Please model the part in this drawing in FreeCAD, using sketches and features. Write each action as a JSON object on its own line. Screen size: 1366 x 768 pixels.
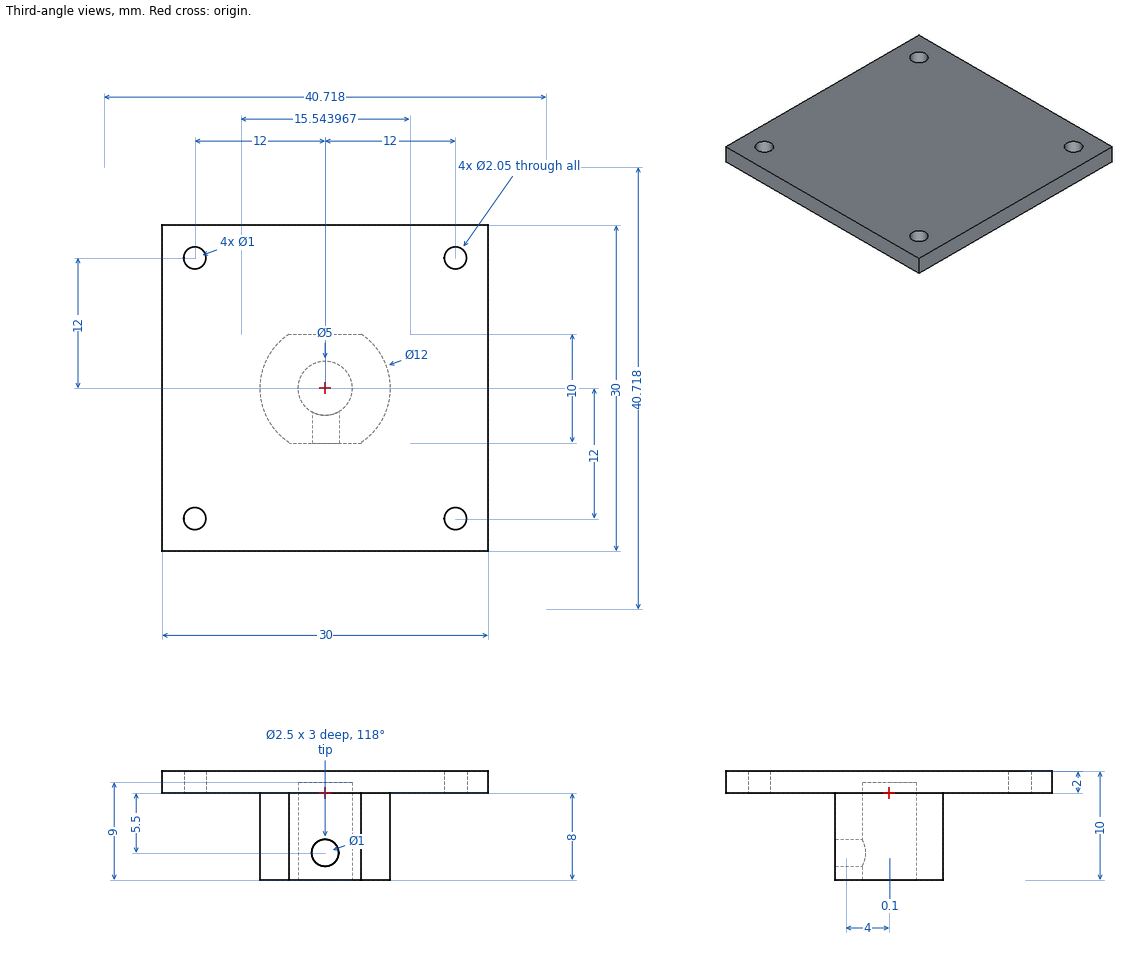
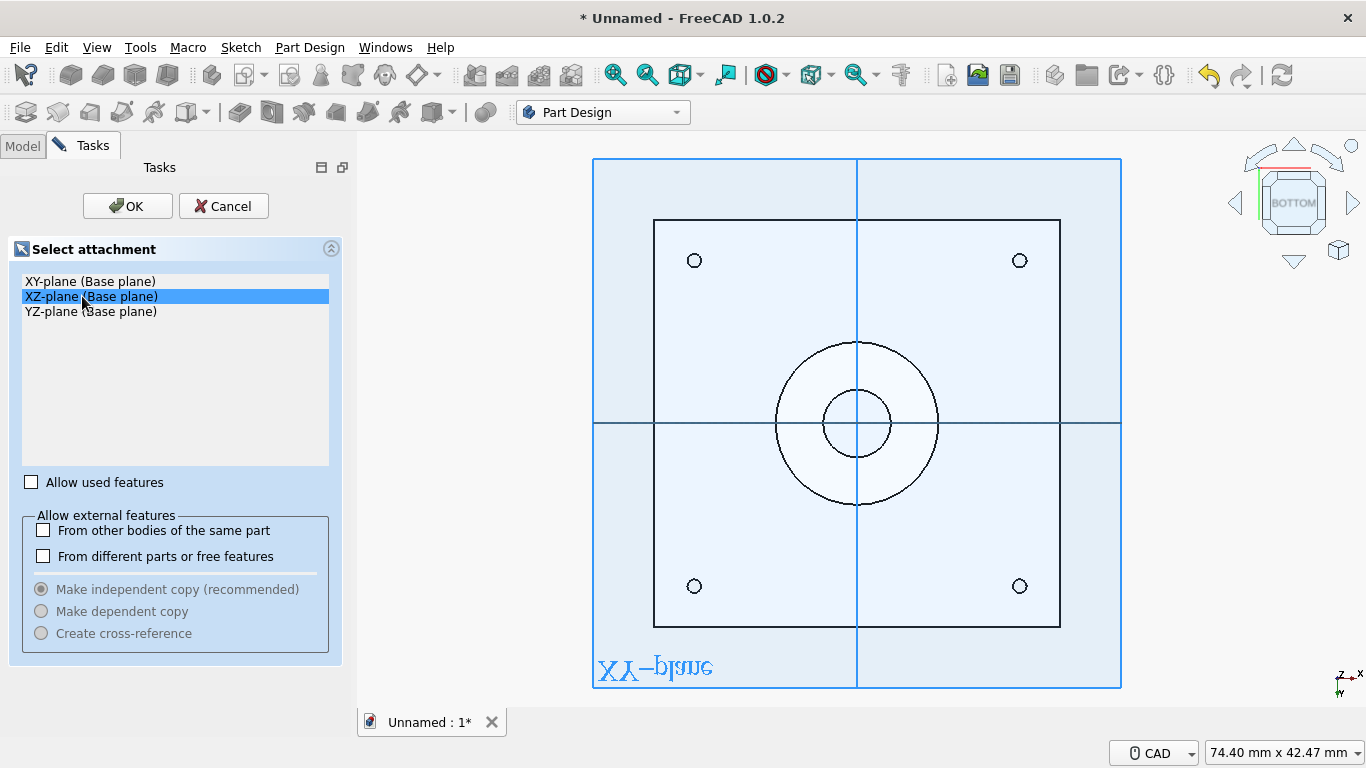
{"action": "left_click", "coordinate": [128, 206]}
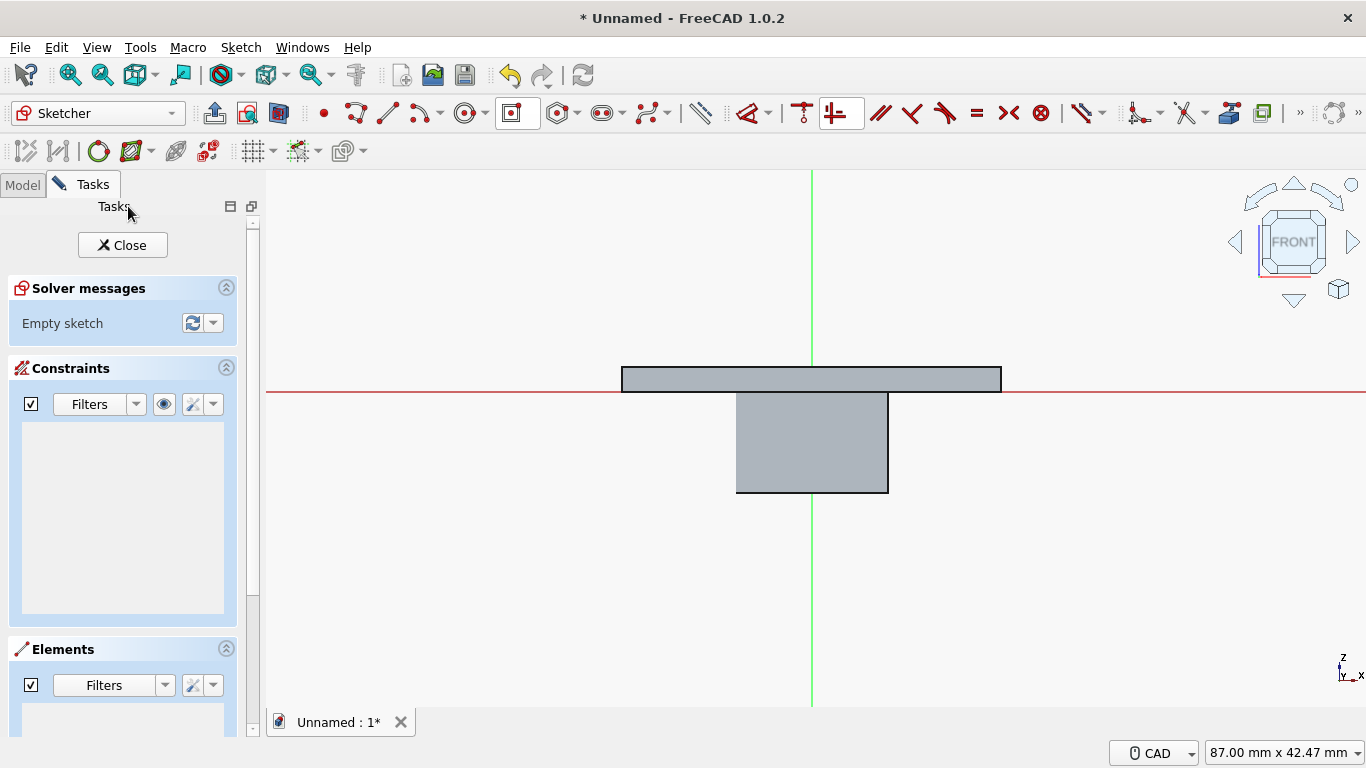
{"action": "key", "text": "q s"}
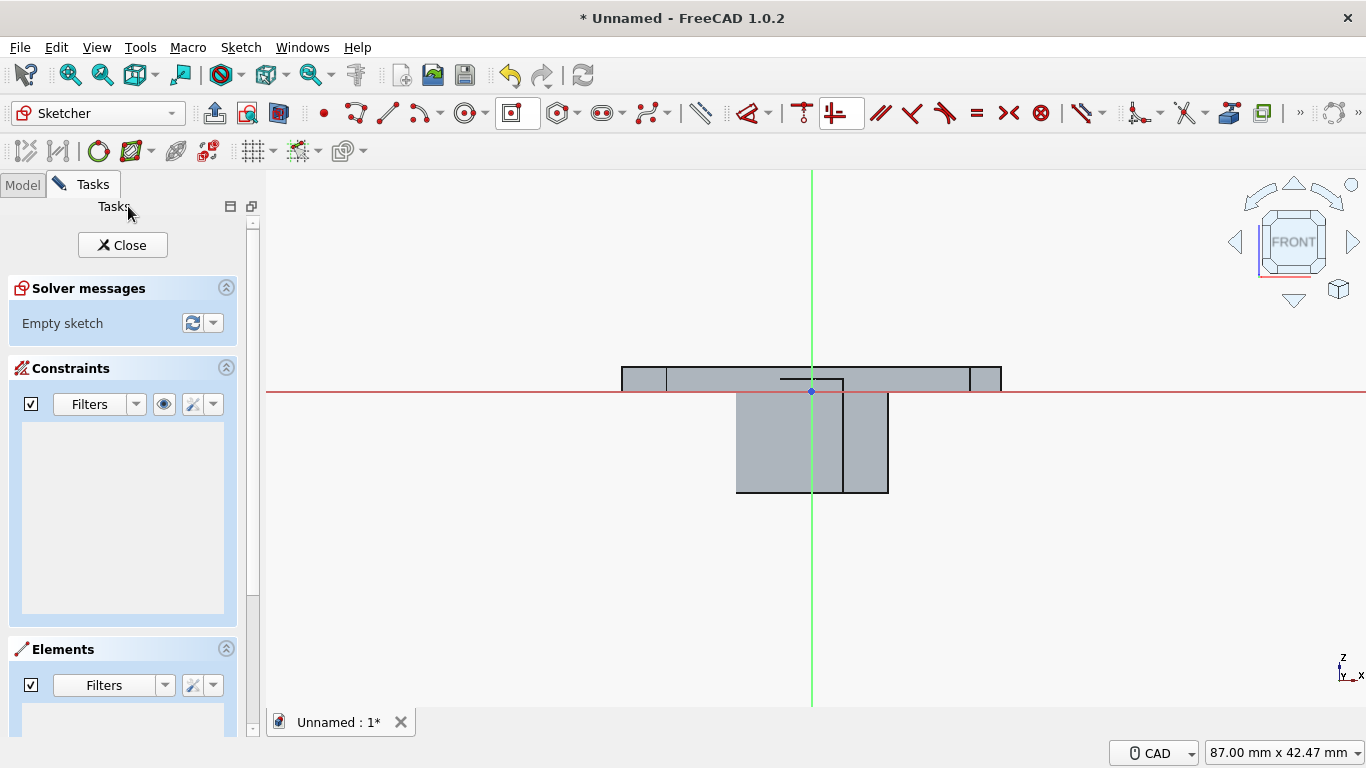
{"action": "scroll", "coordinate": [815, 463], "scroll_direction": "up", "scroll_amount": 15}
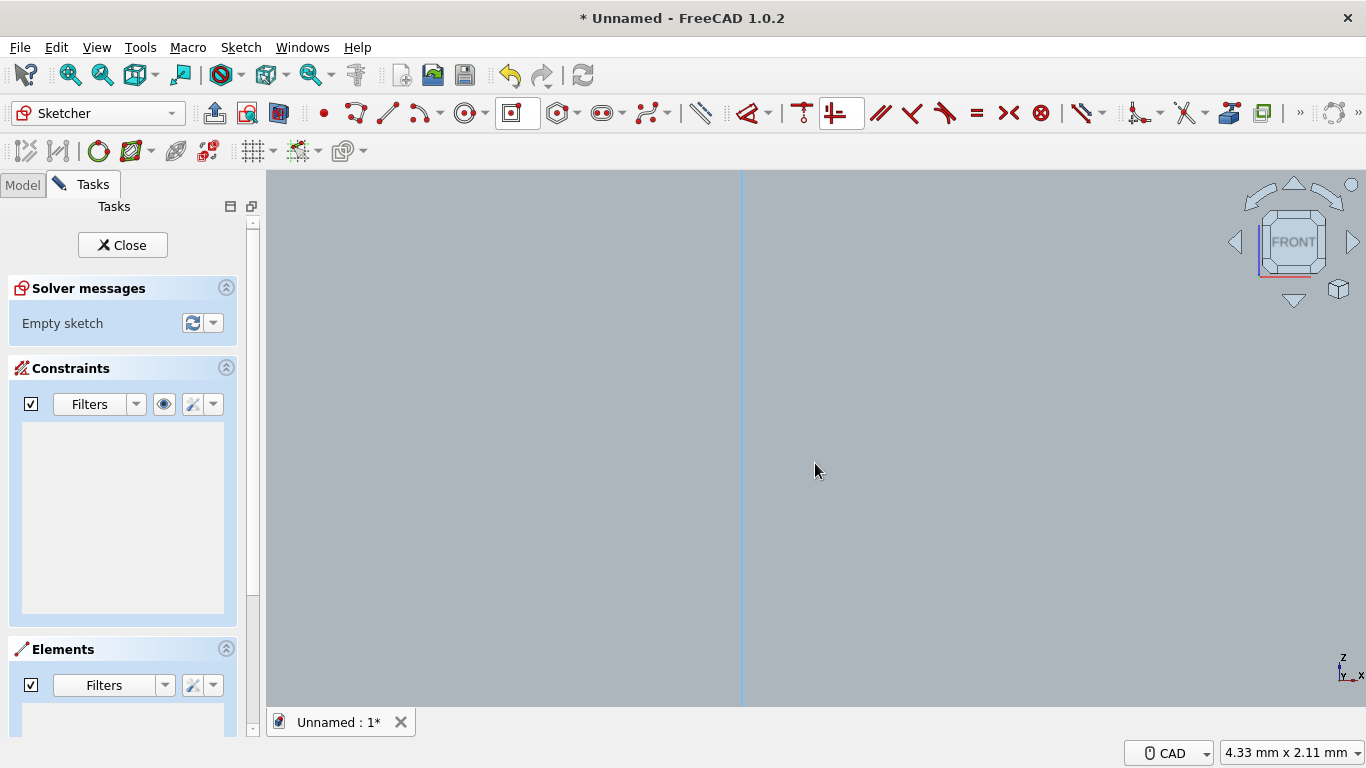
{"action": "key", "text": "g c"}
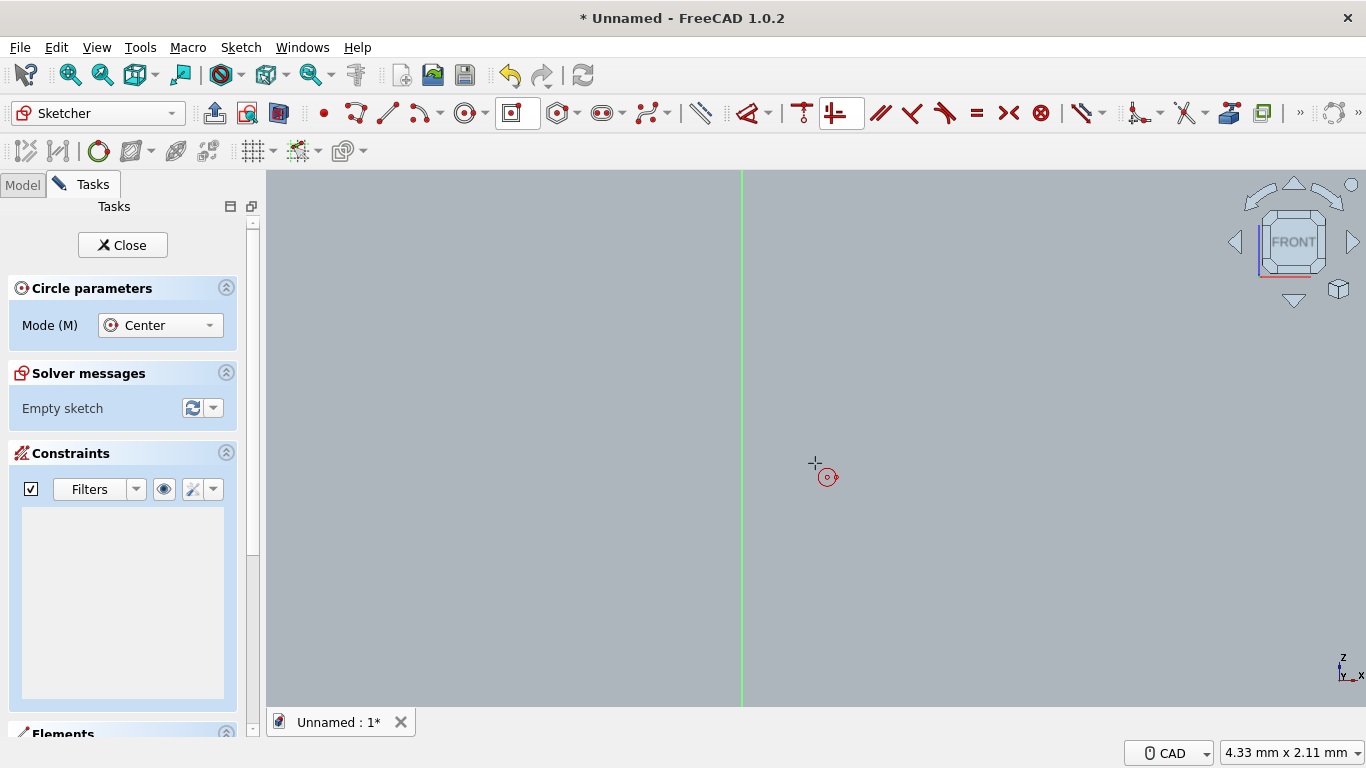
{"action": "left_click", "coordinate": [742, 421]}
{"action": "left_click", "coordinate": [832, 331]}
{"action": "key", "text": "Escape"}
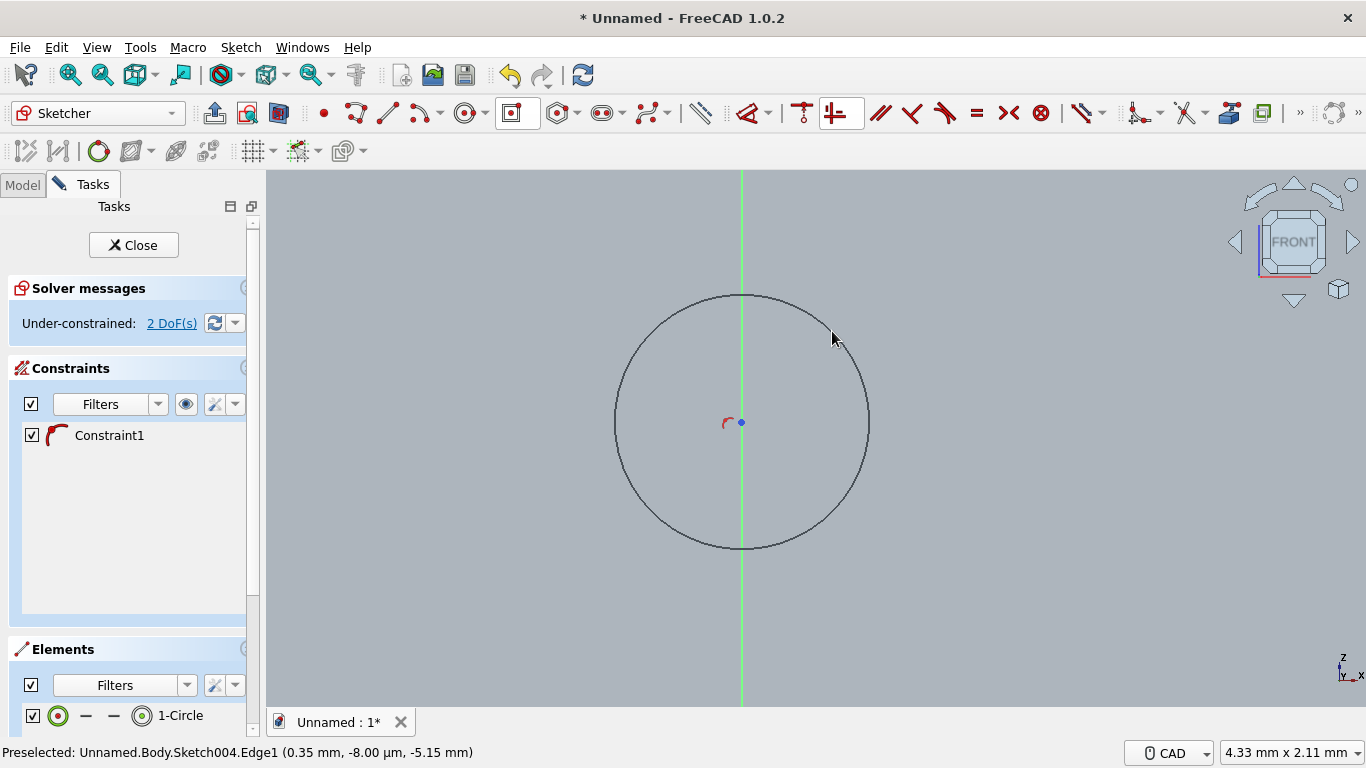
{"action": "left_click", "coordinate": [748, 114]}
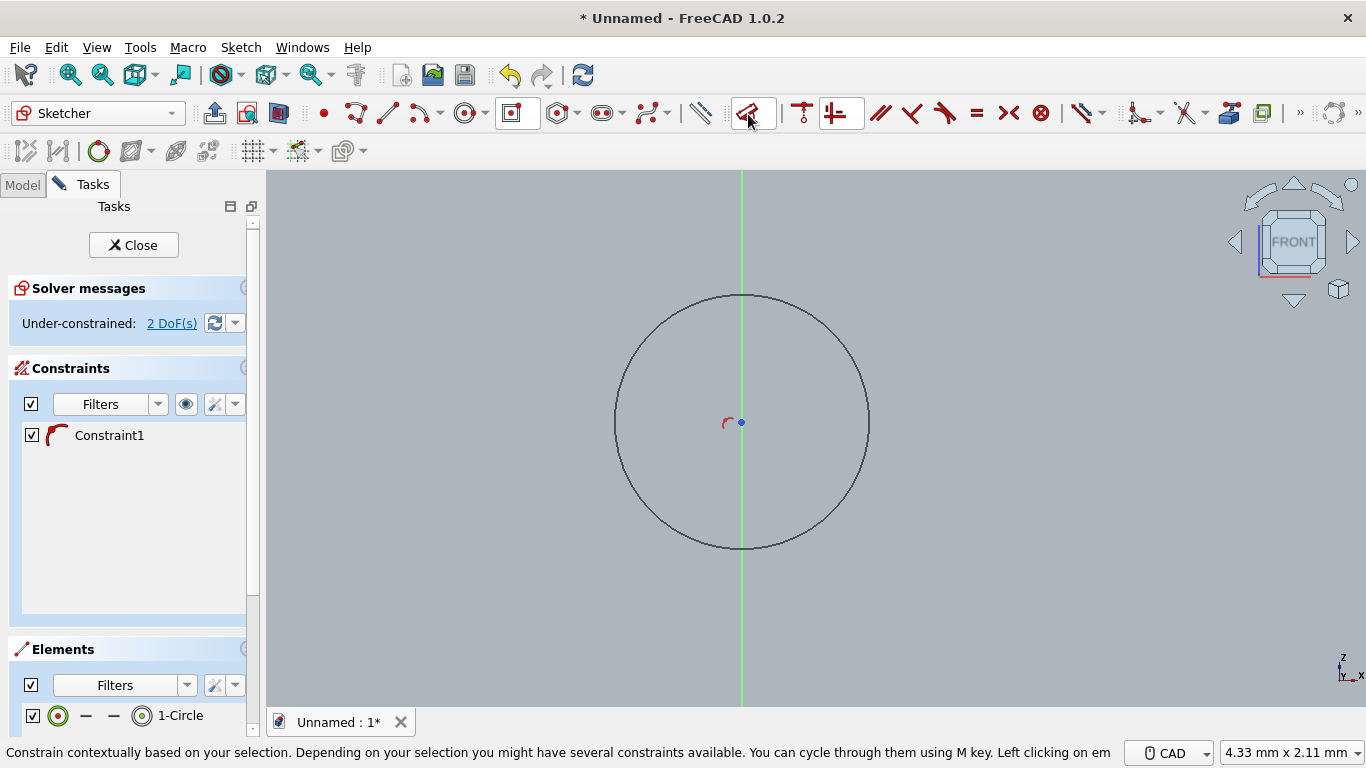
{"action": "left_click", "coordinate": [832, 332]}
{"action": "left_click", "coordinate": [855, 309]}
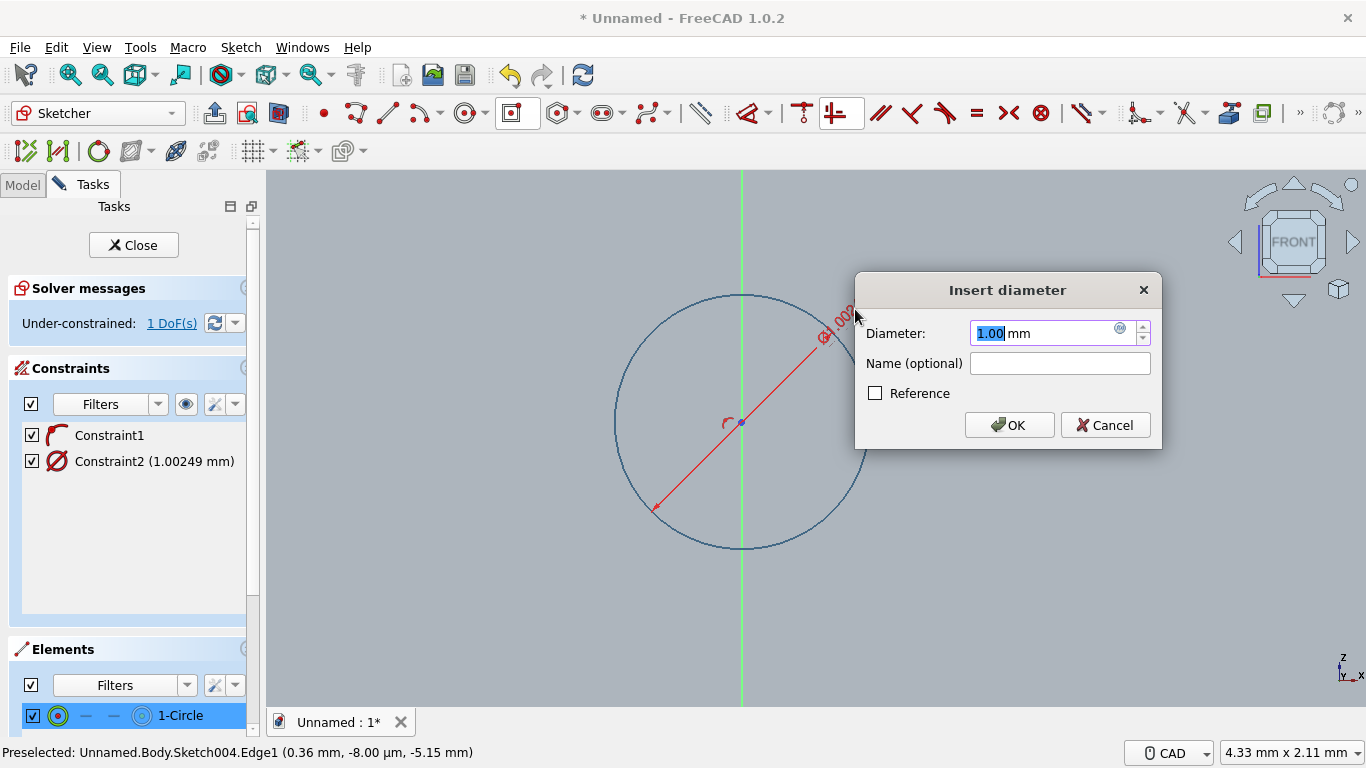
{"action": "type", "text": "1"}
{"action": "key", "text": "Return"}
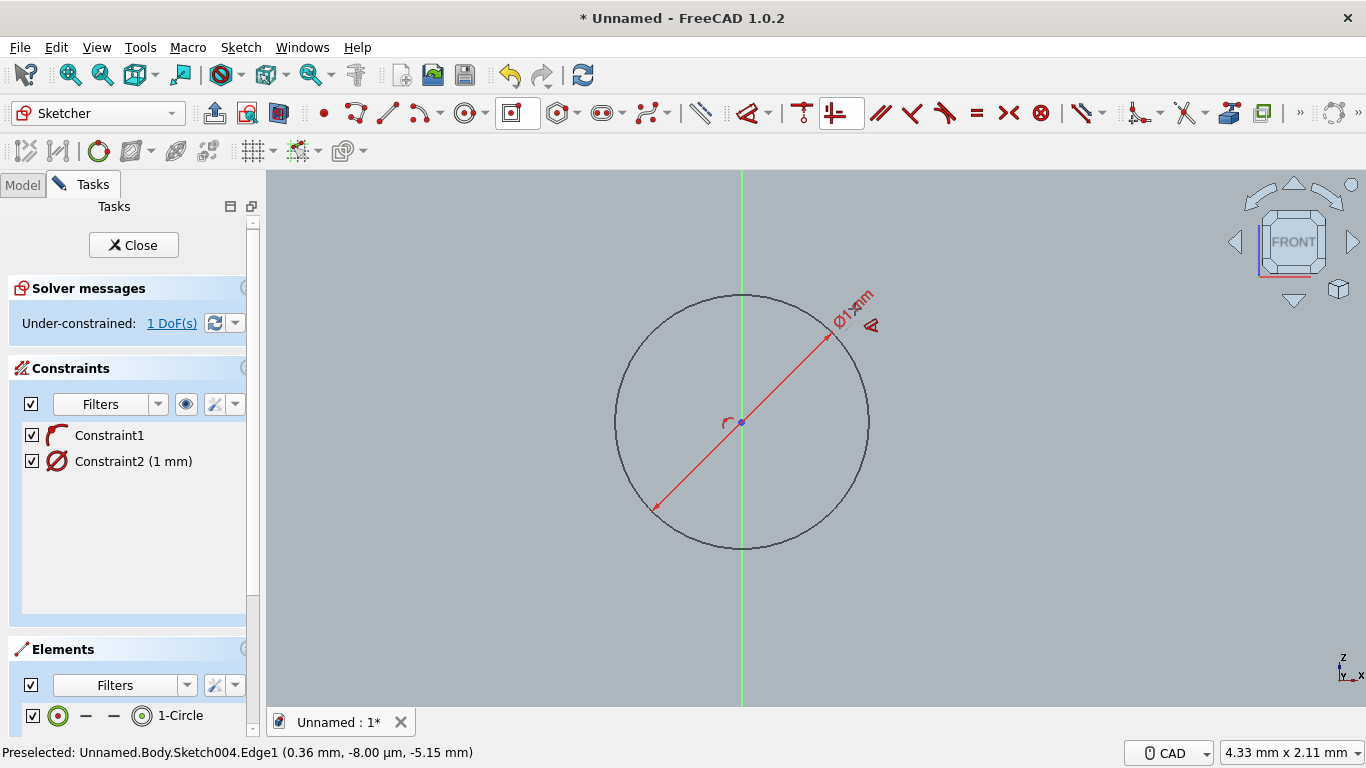
{"action": "left_click", "coordinate": [742, 422]}
{"action": "left_click", "coordinate": [776, 258]}